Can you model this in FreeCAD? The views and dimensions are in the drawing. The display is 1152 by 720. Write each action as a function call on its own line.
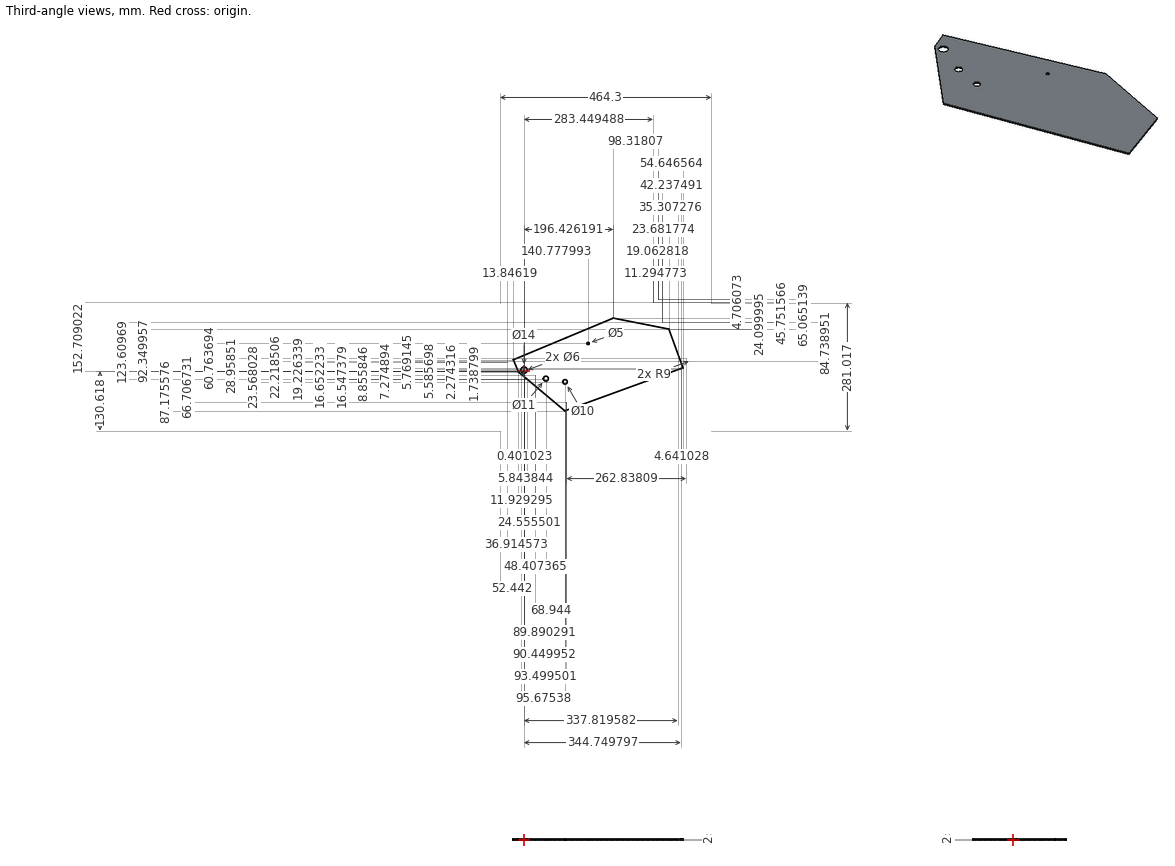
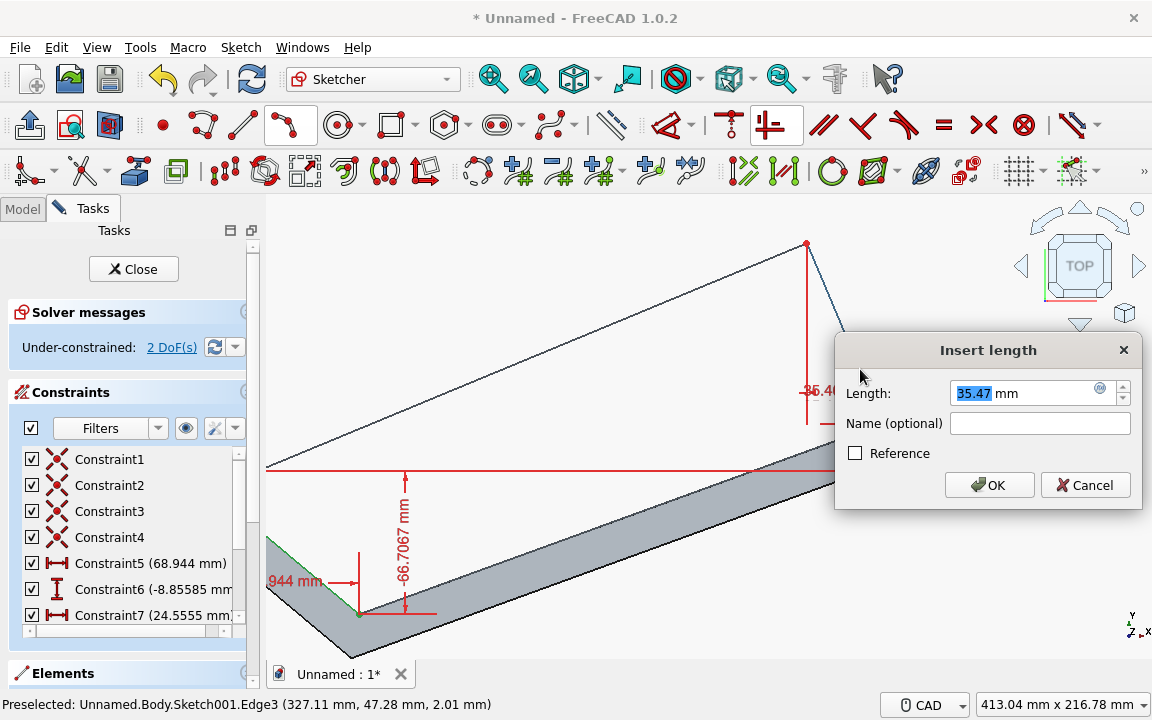
text(35.307276)
key(Return)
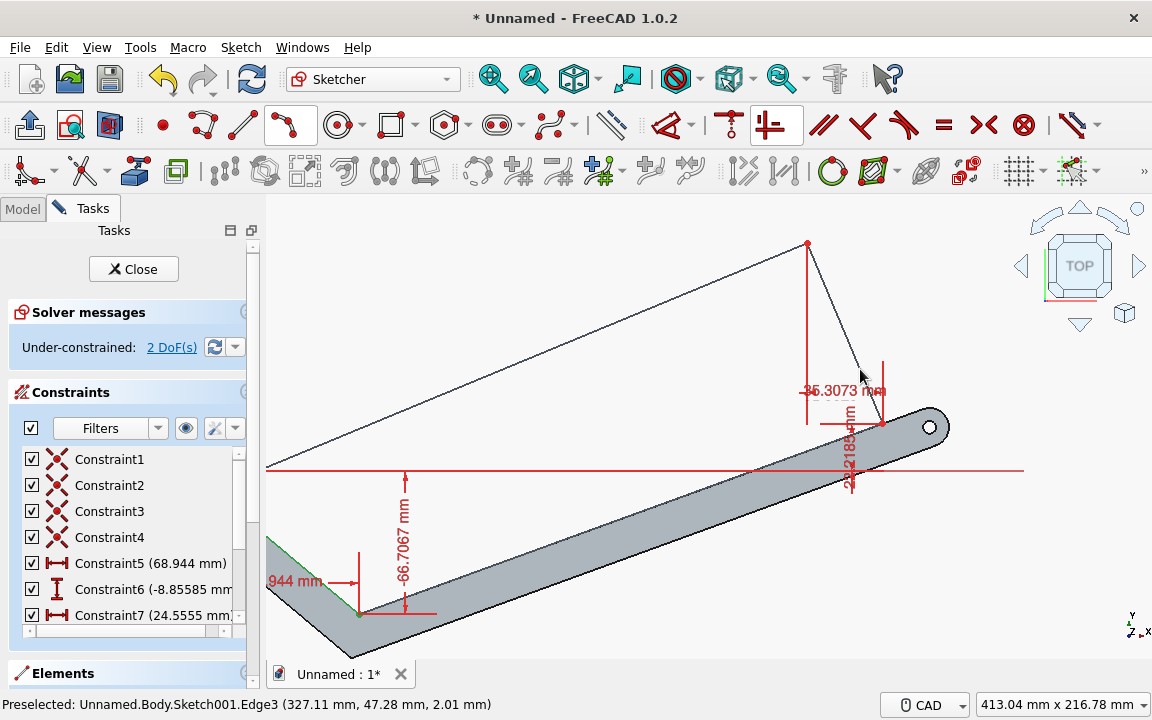
click(860, 369)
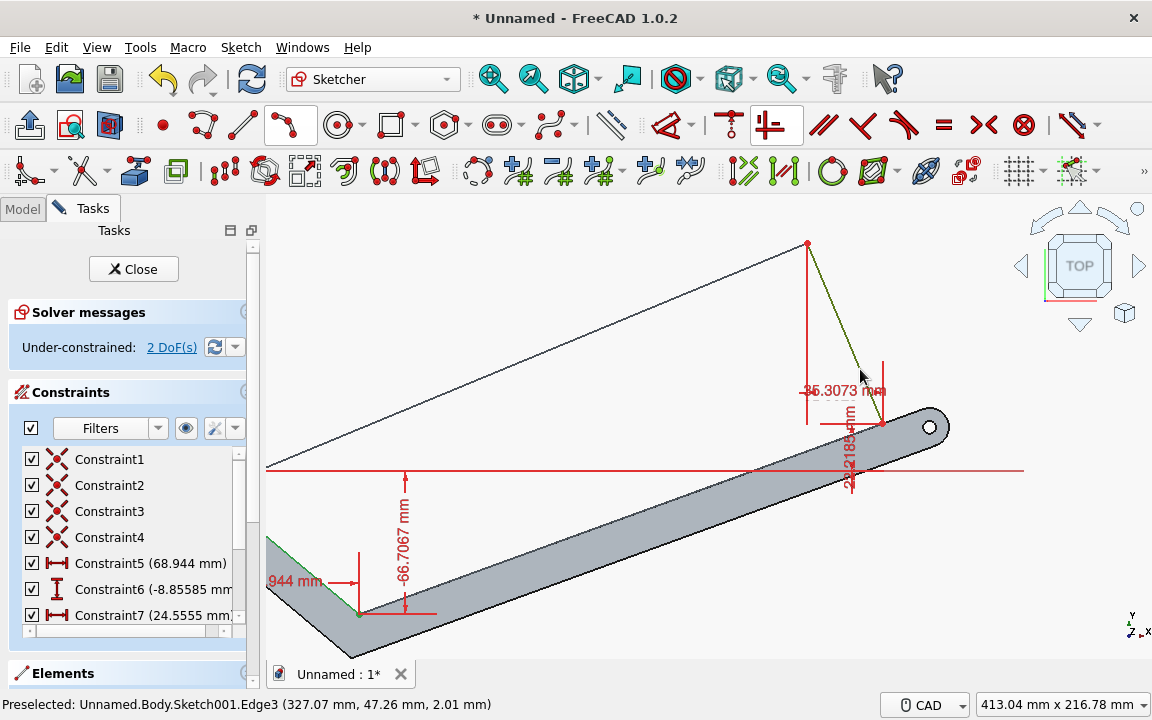
key(i)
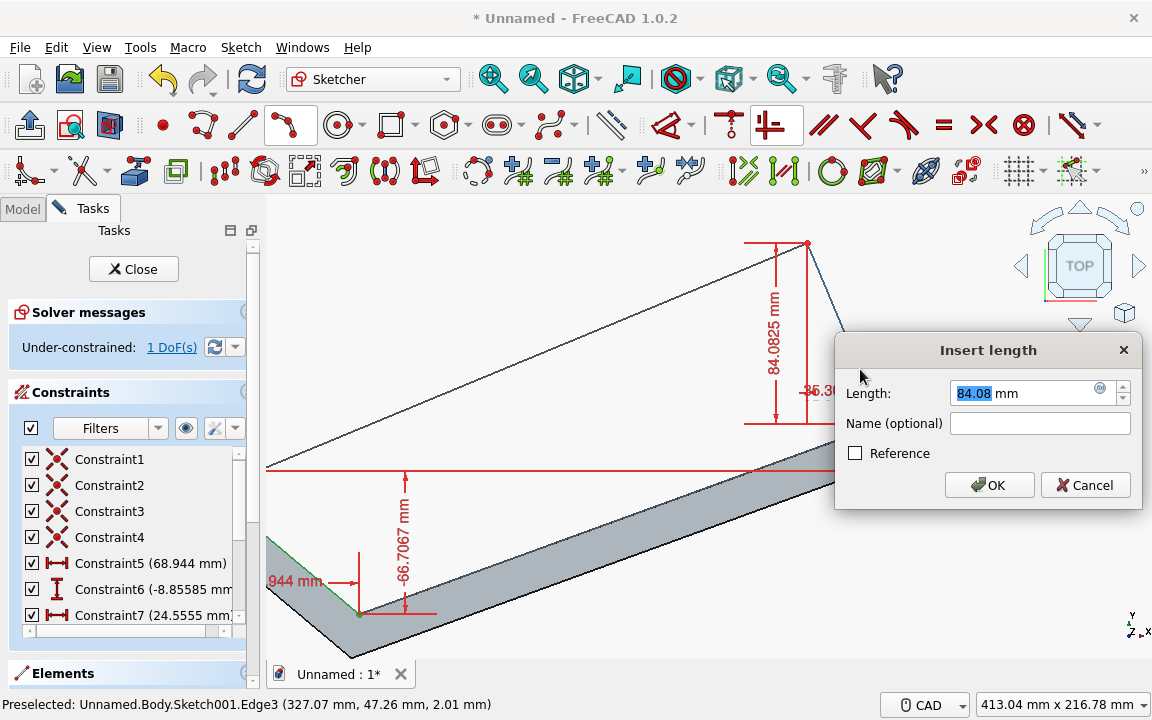
text(84.738951)
key(Return)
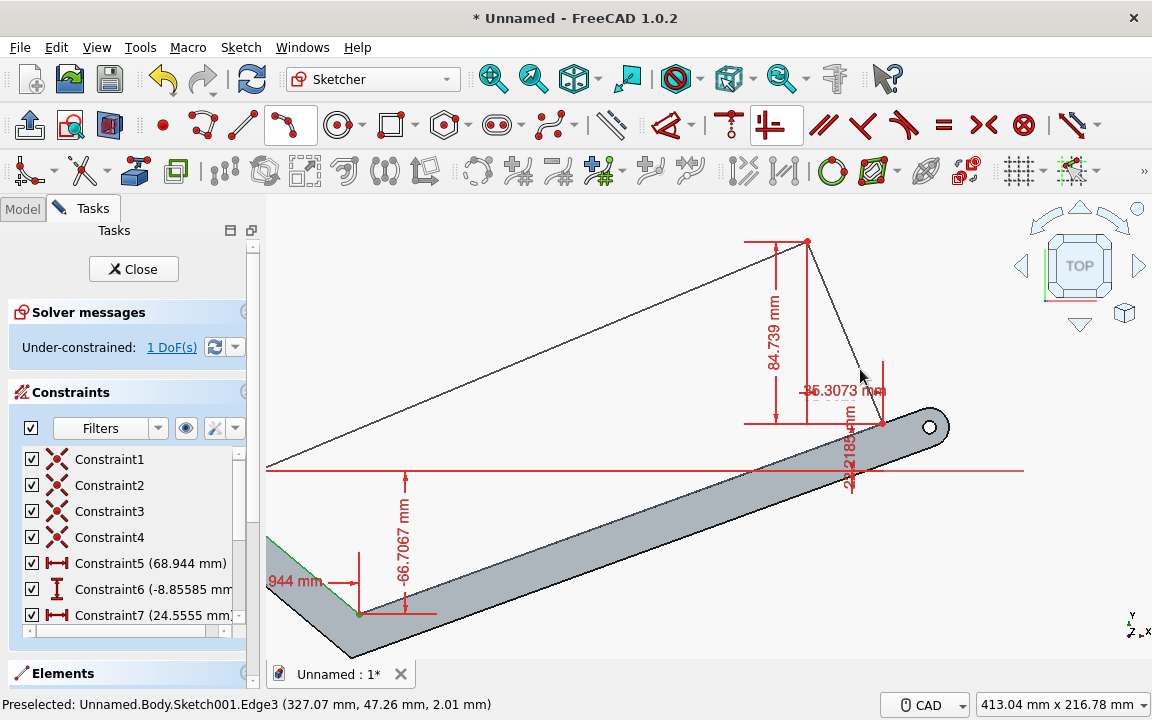
click(883, 424)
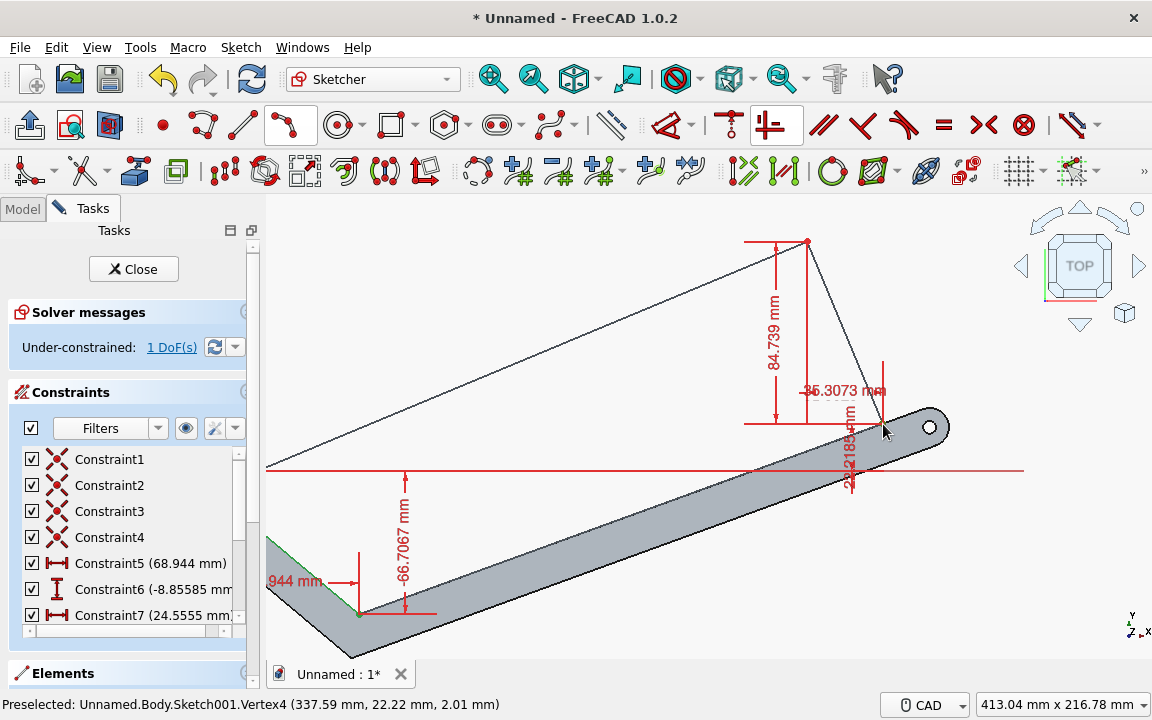
key(l)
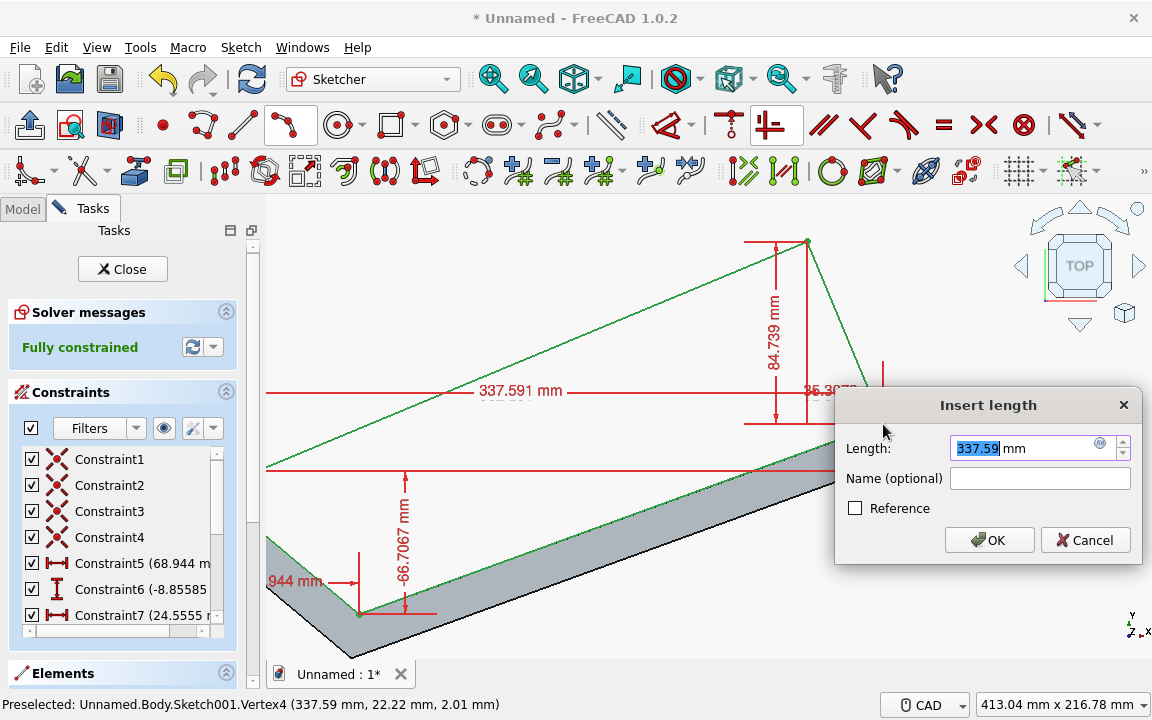
text(337.819582)
key(Return)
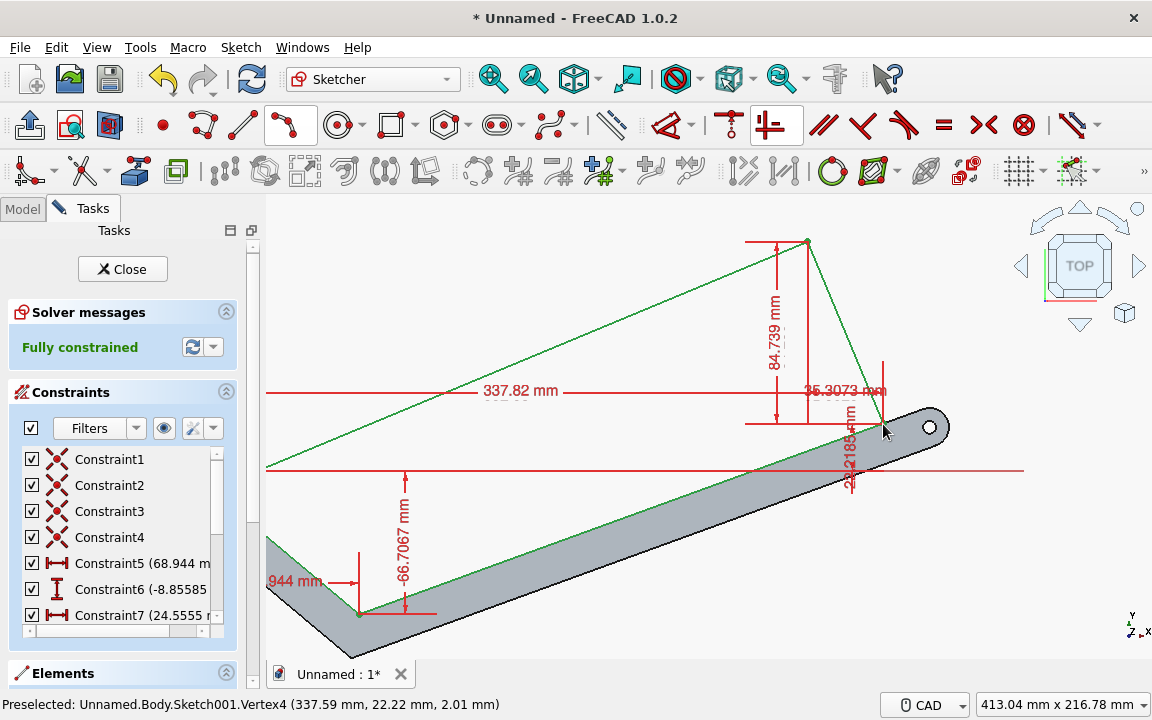
click(123, 269)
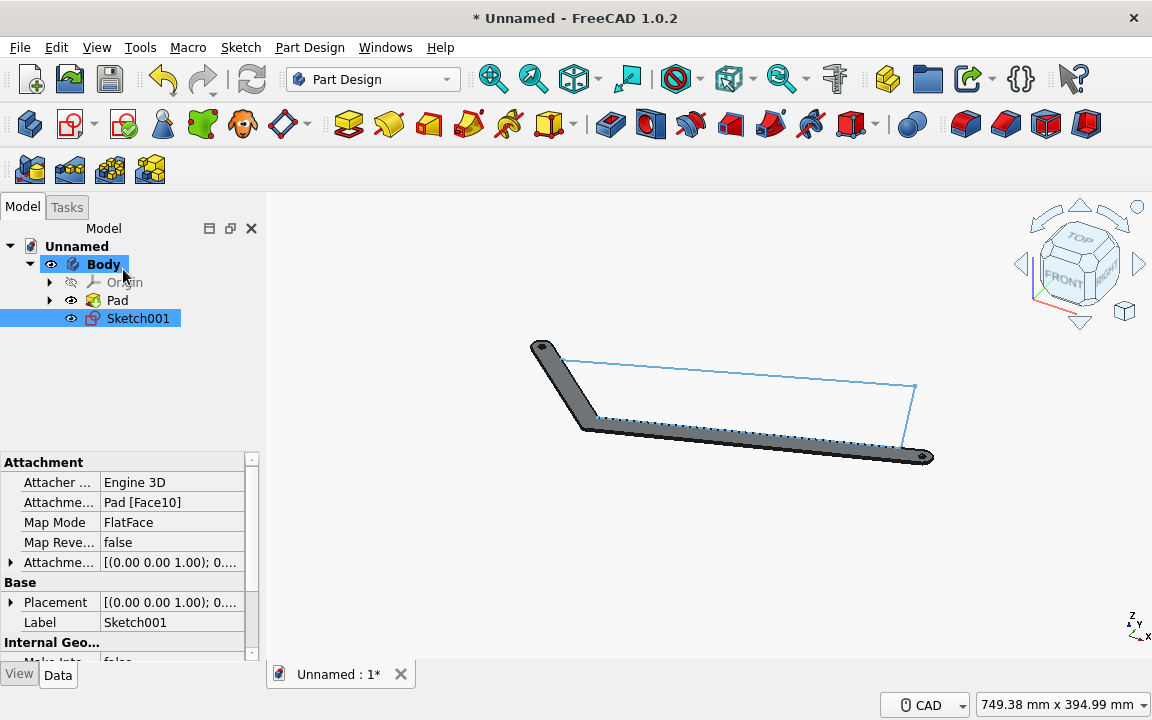
click(350, 124)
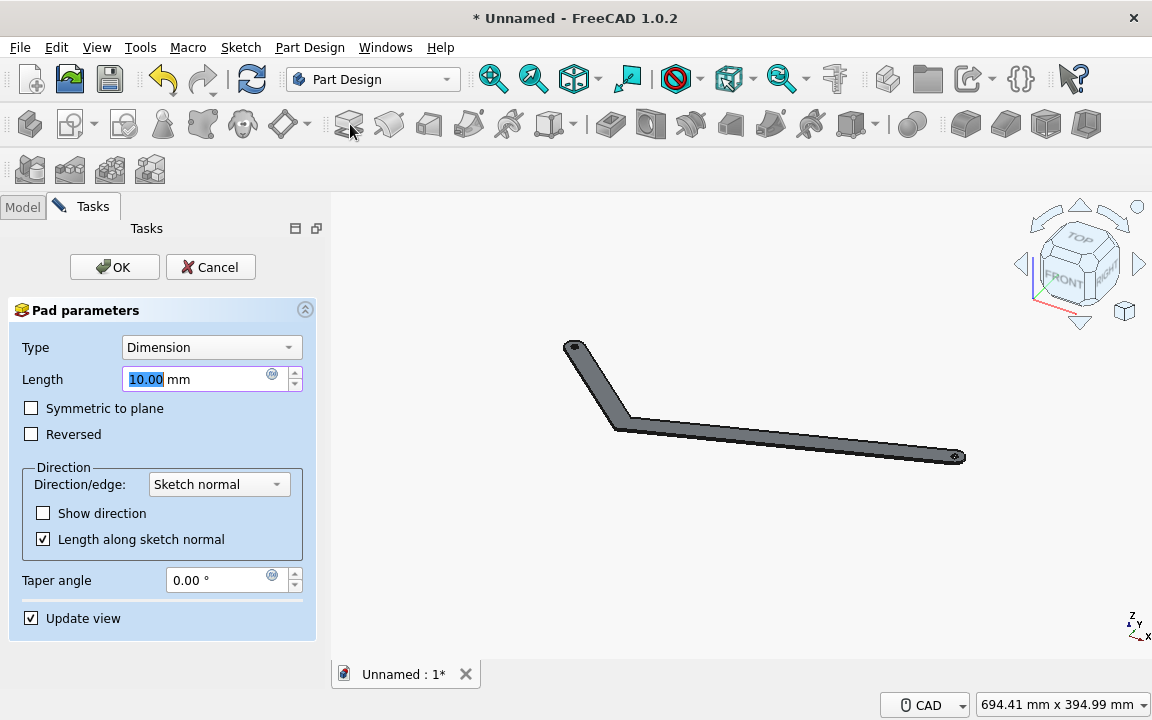
text(2)
key(Tab)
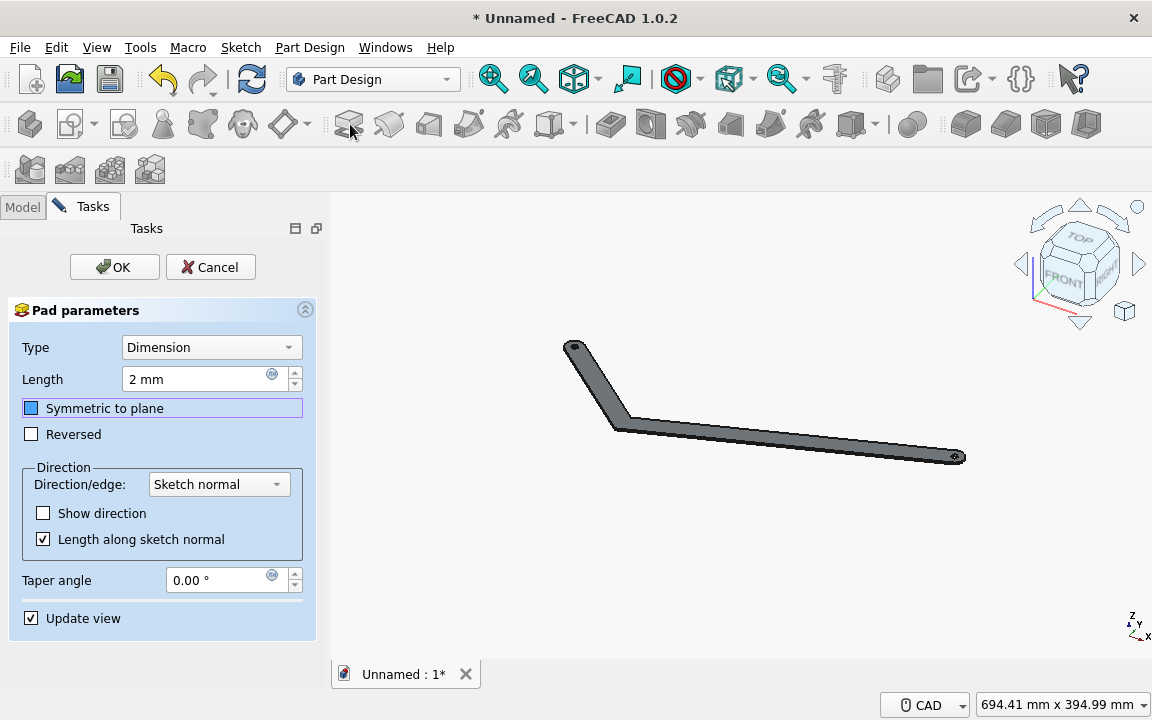
click(30, 434)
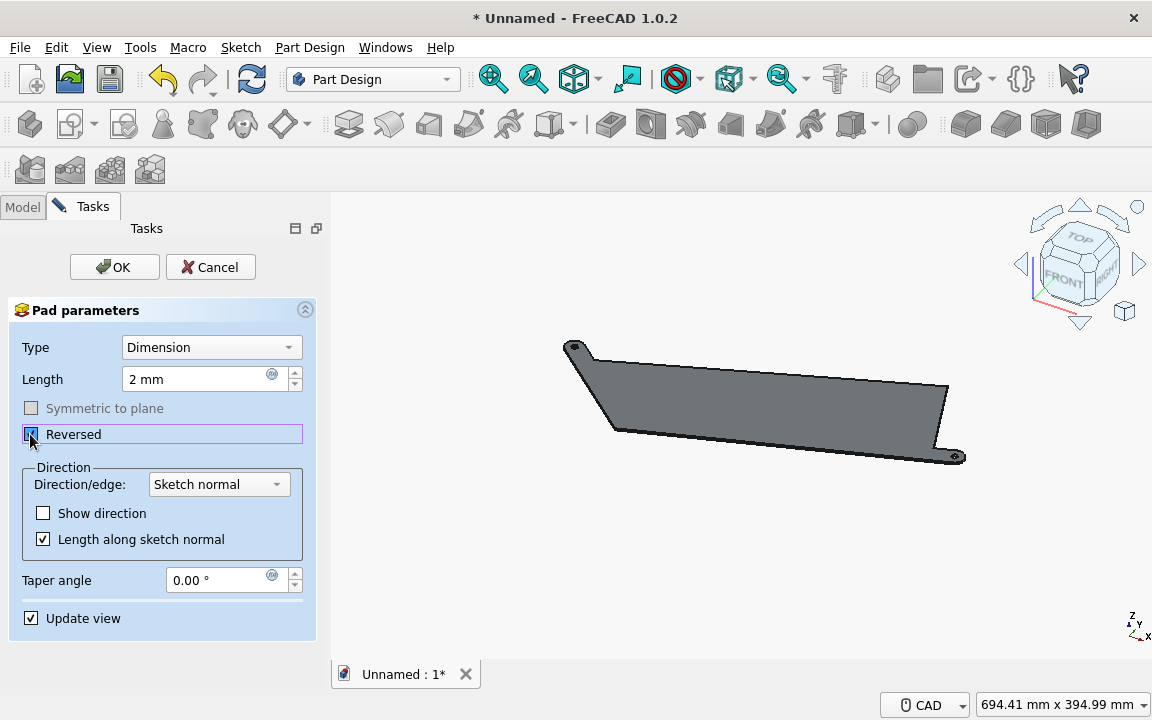
click(115, 267)